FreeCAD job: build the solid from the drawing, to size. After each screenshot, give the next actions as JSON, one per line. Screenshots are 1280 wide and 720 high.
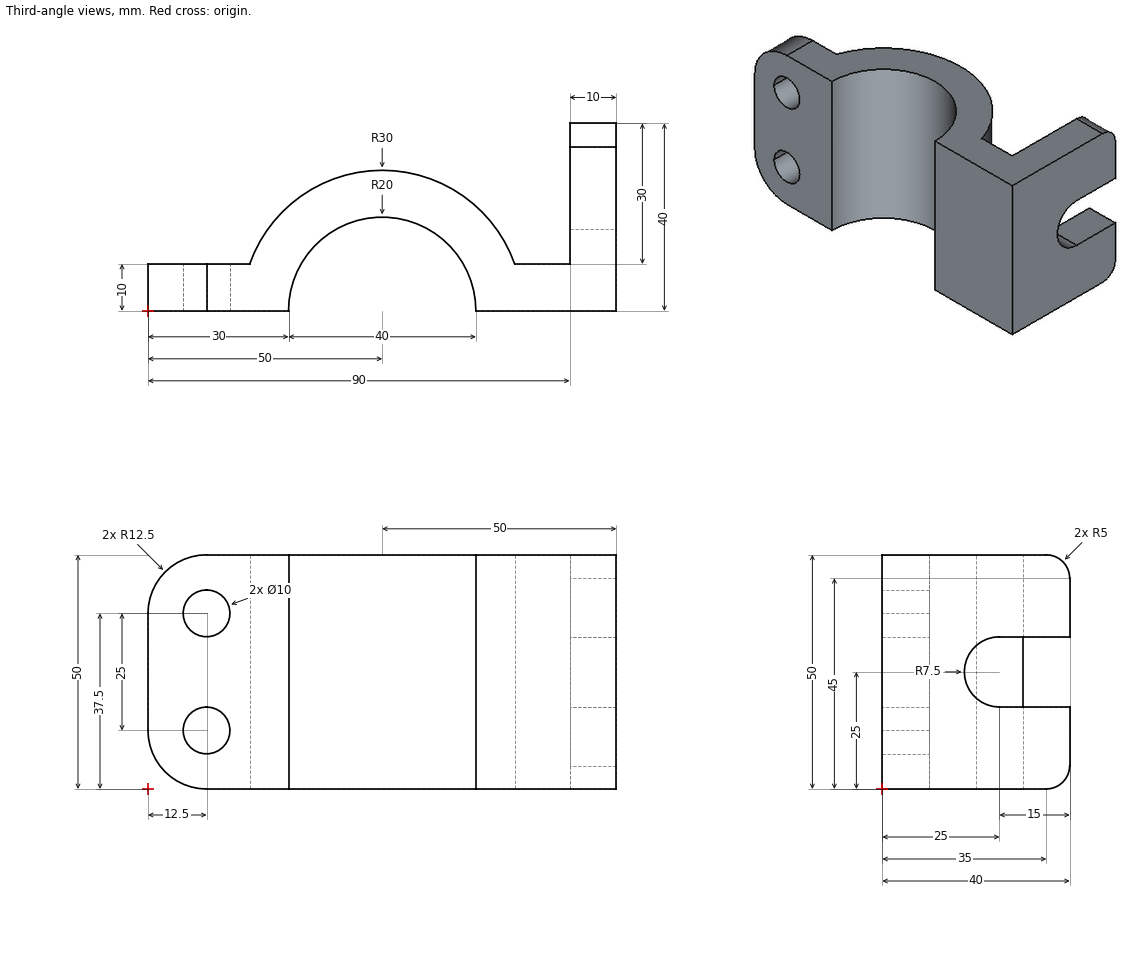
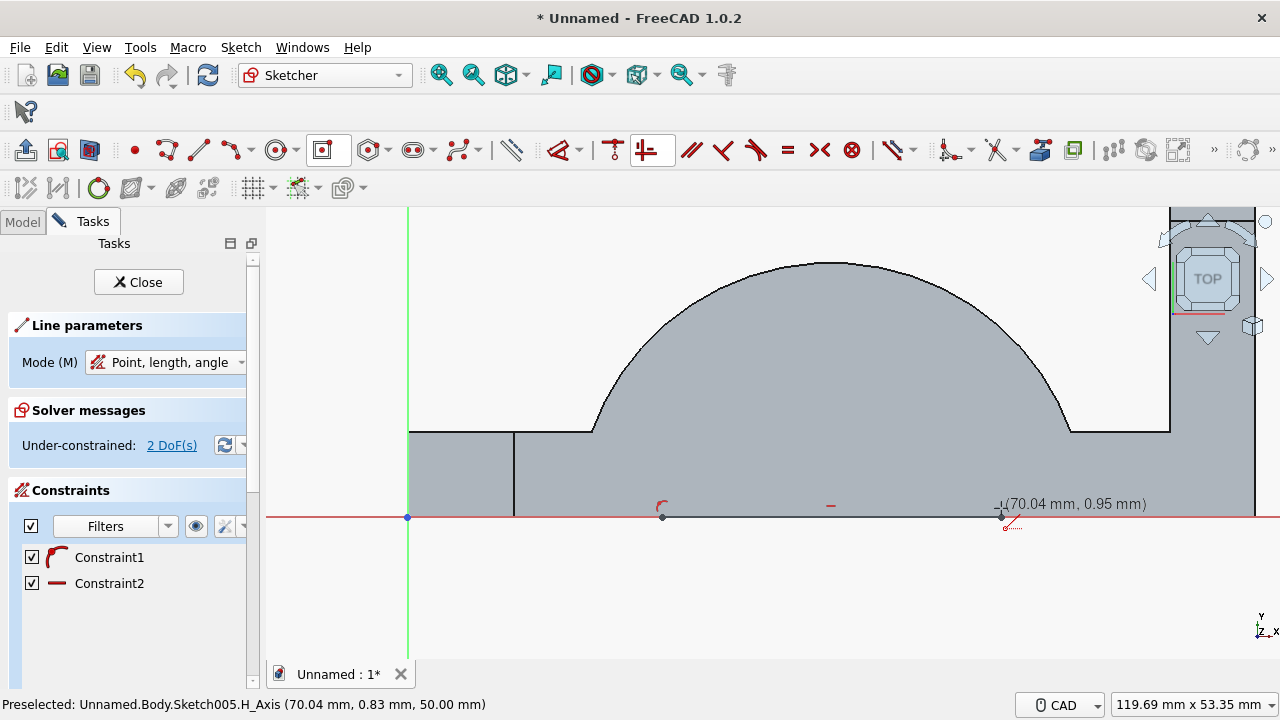
{"action": "left_click", "coordinate": [232, 150]}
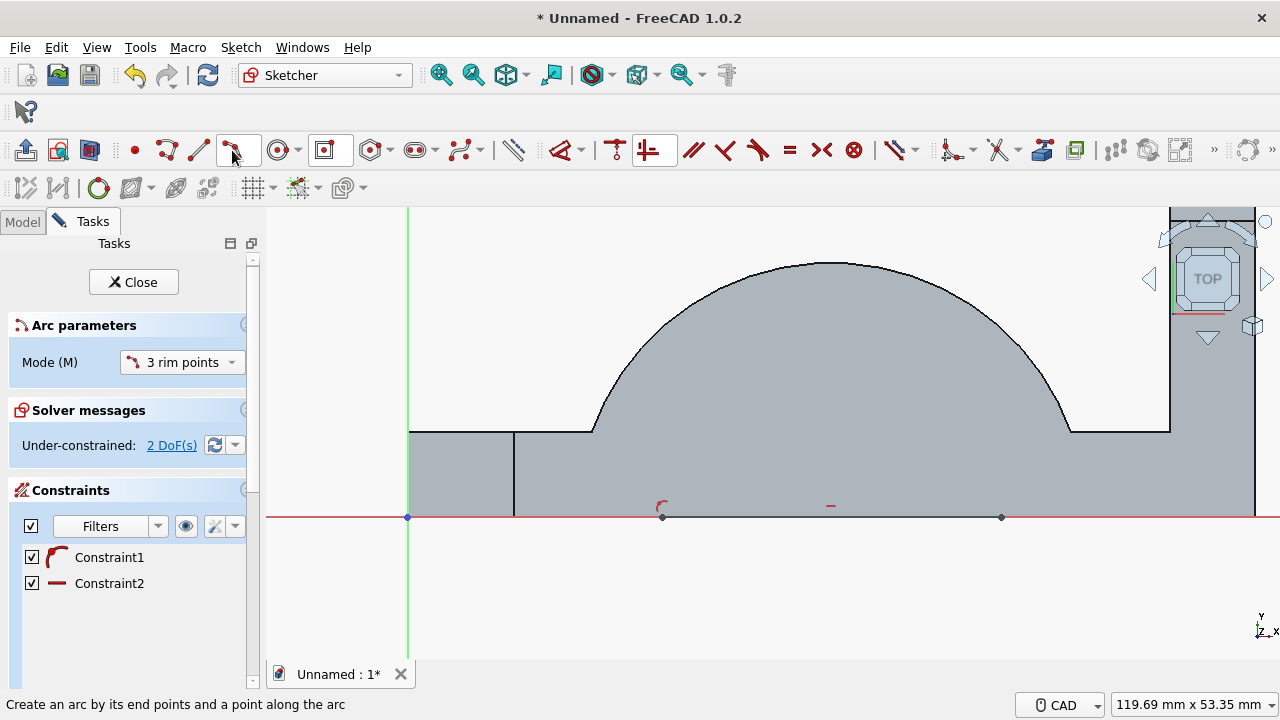
{"action": "left_click", "coordinate": [1001, 508]}
{"action": "left_click", "coordinate": [662, 517]}
{"action": "left_click", "coordinate": [831, 348]}
{"action": "key", "text": "Escape"}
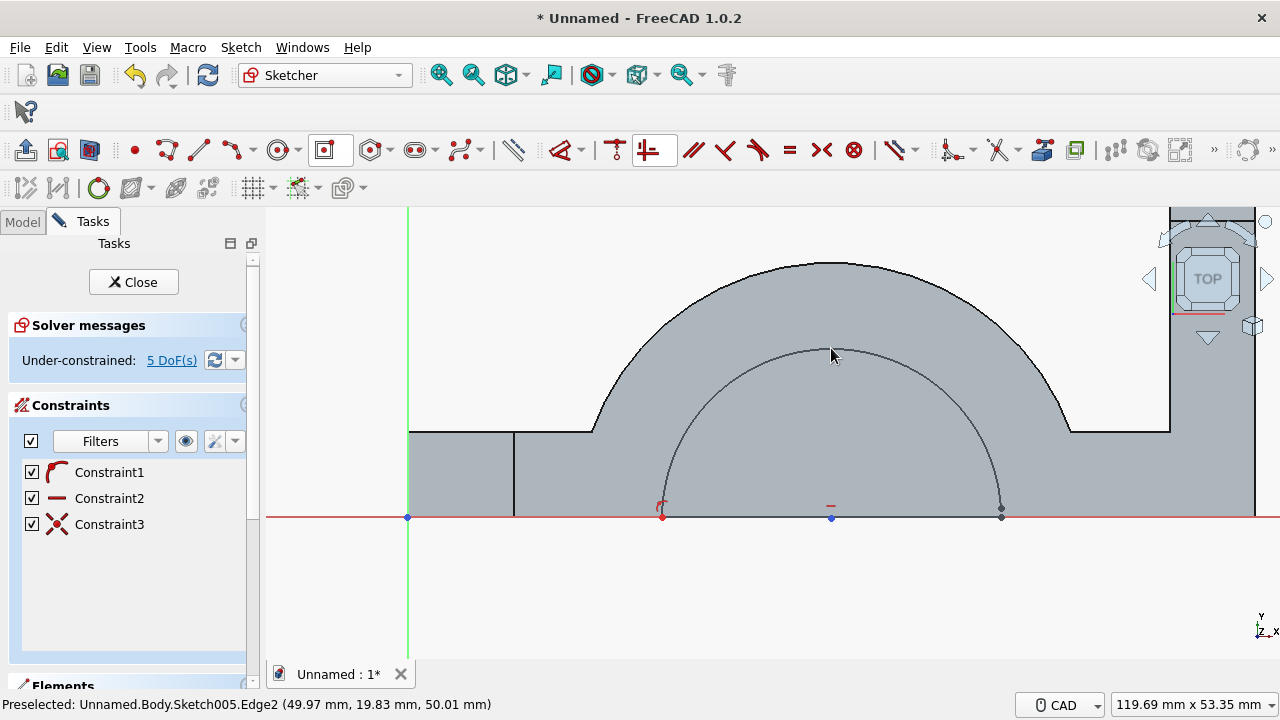
{"action": "left_click", "coordinate": [832, 519]}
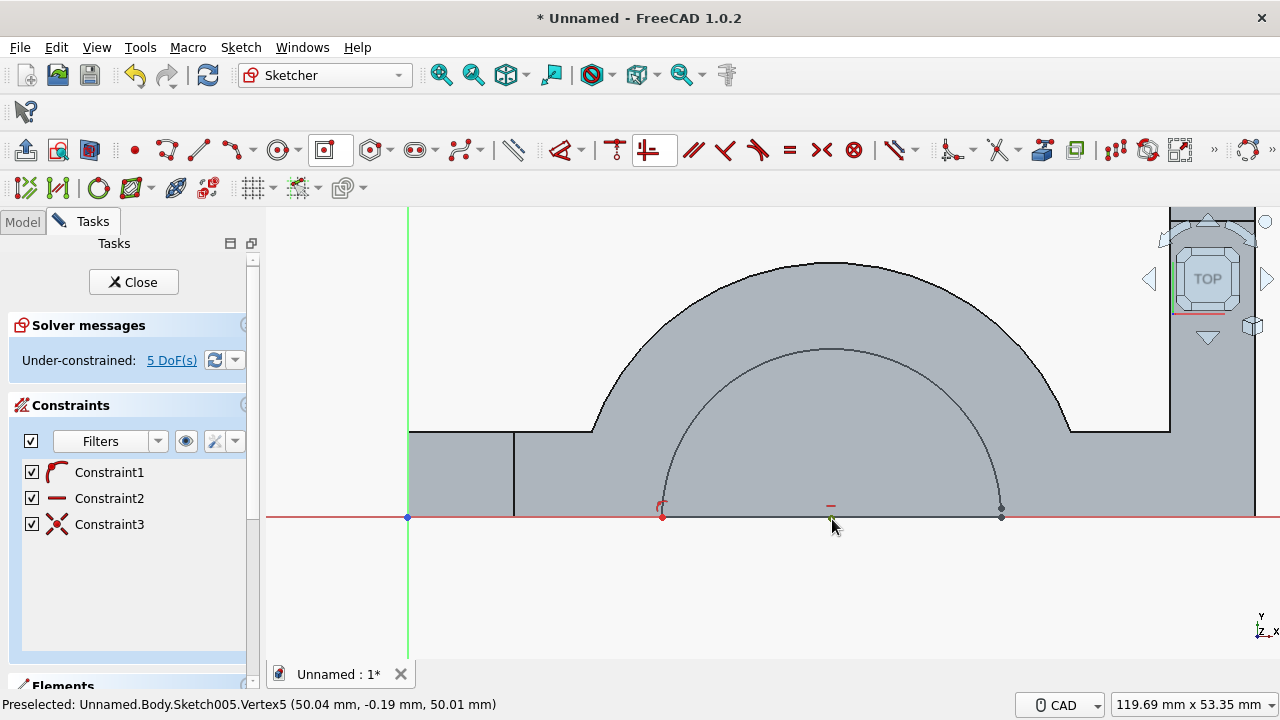
{"action": "left_click", "coordinate": [353, 517]}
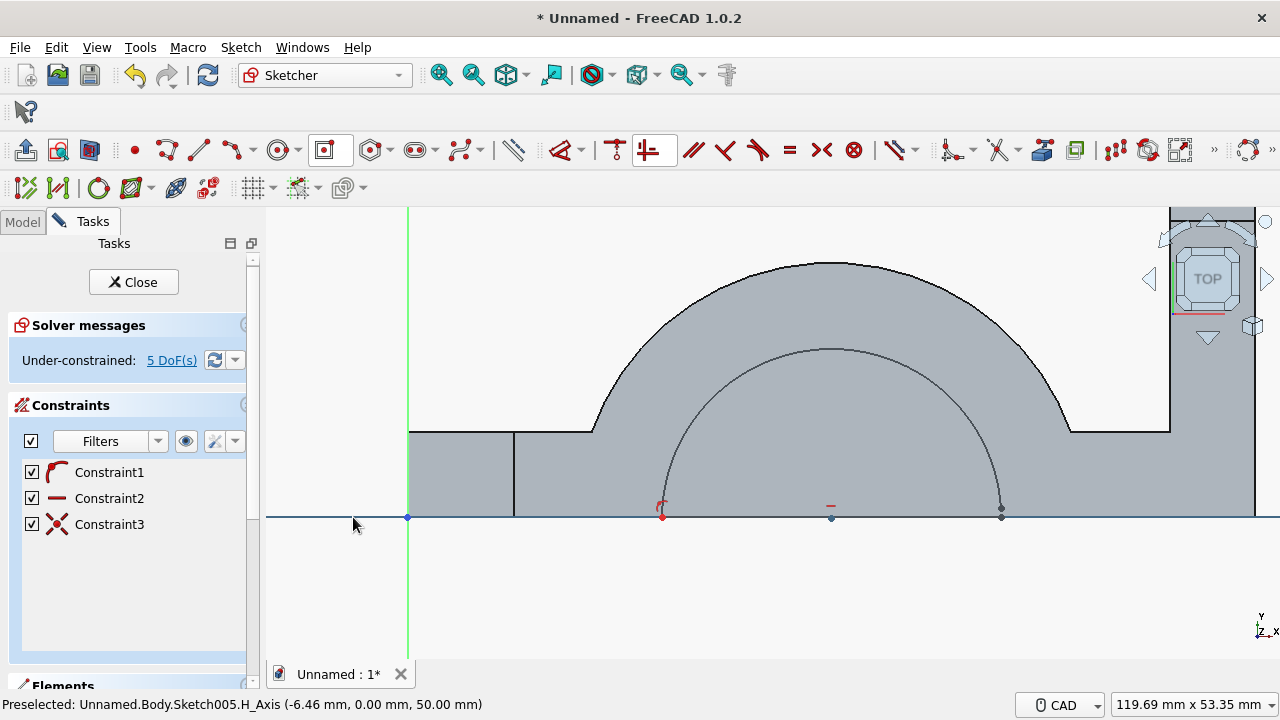
{"action": "left_click", "coordinate": [616, 150]}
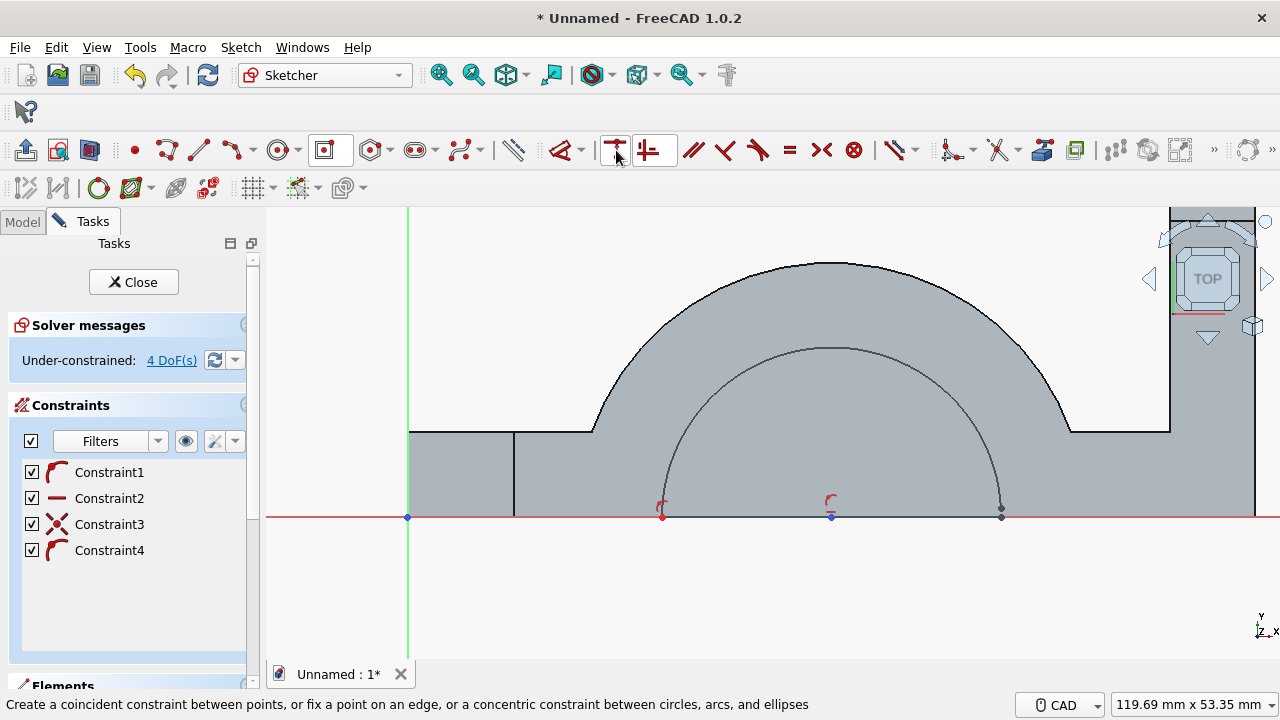
{"action": "left_click", "coordinate": [560, 150]}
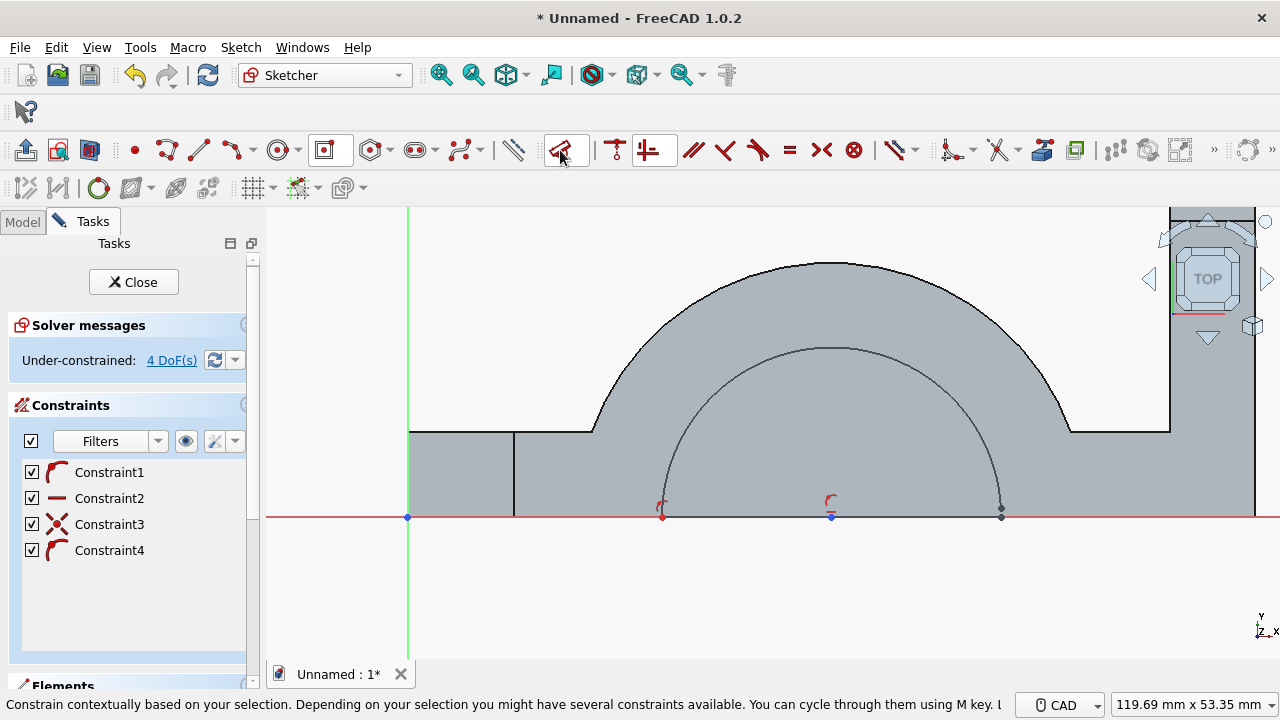
{"action": "left_click", "coordinate": [927, 377]}
{"action": "left_click", "coordinate": [945, 351]}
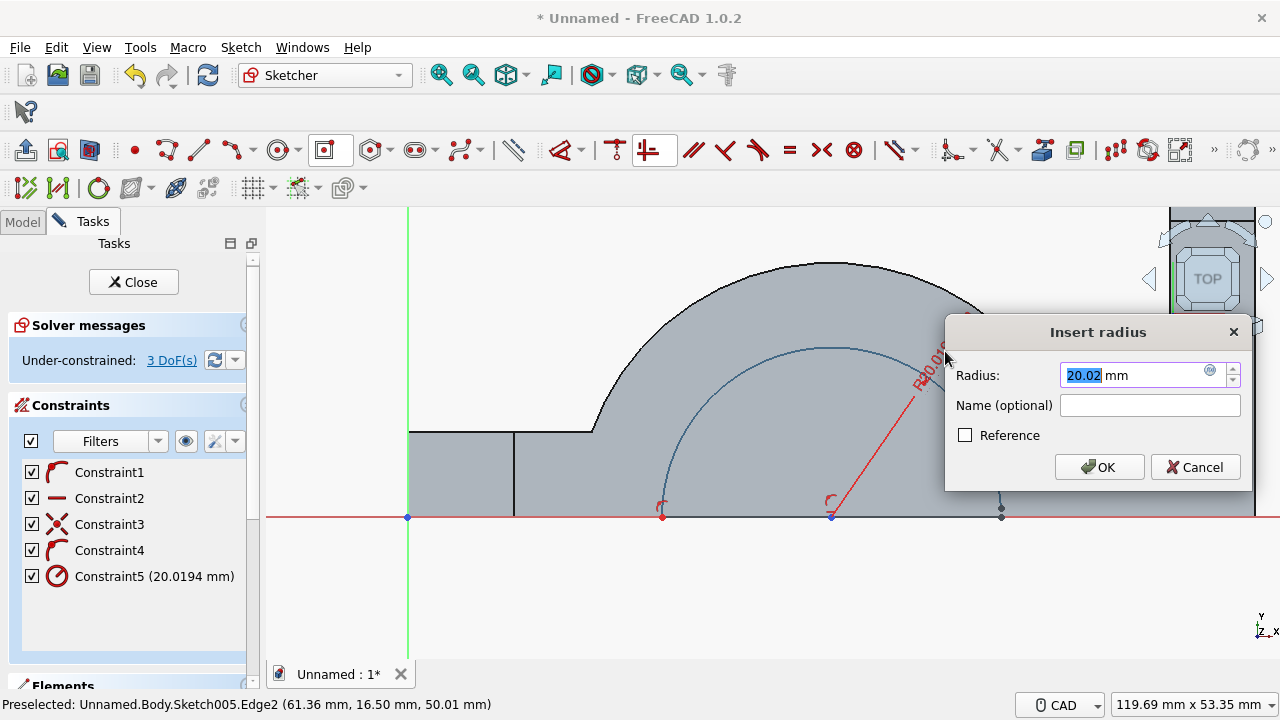
{"action": "type", "text": "20"}
{"action": "key", "text": "Return"}
{"action": "key", "text": "Escape"}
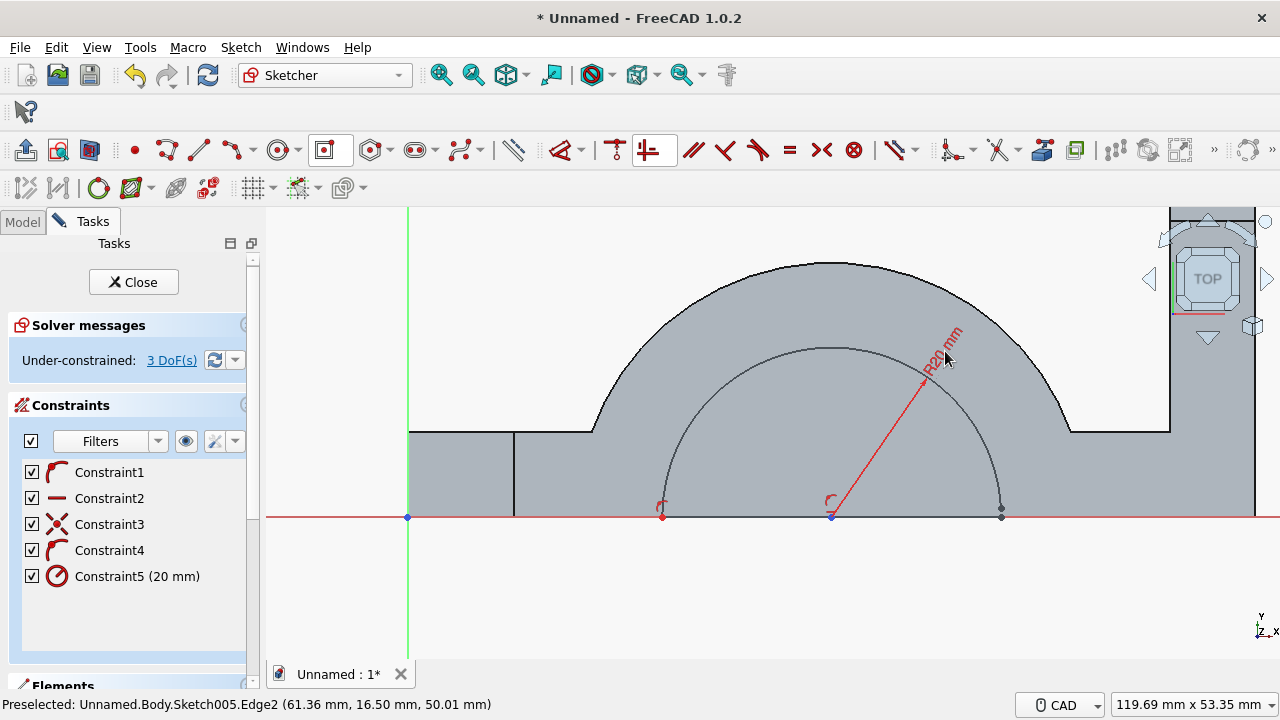
{"action": "left_click", "coordinate": [1001, 509]}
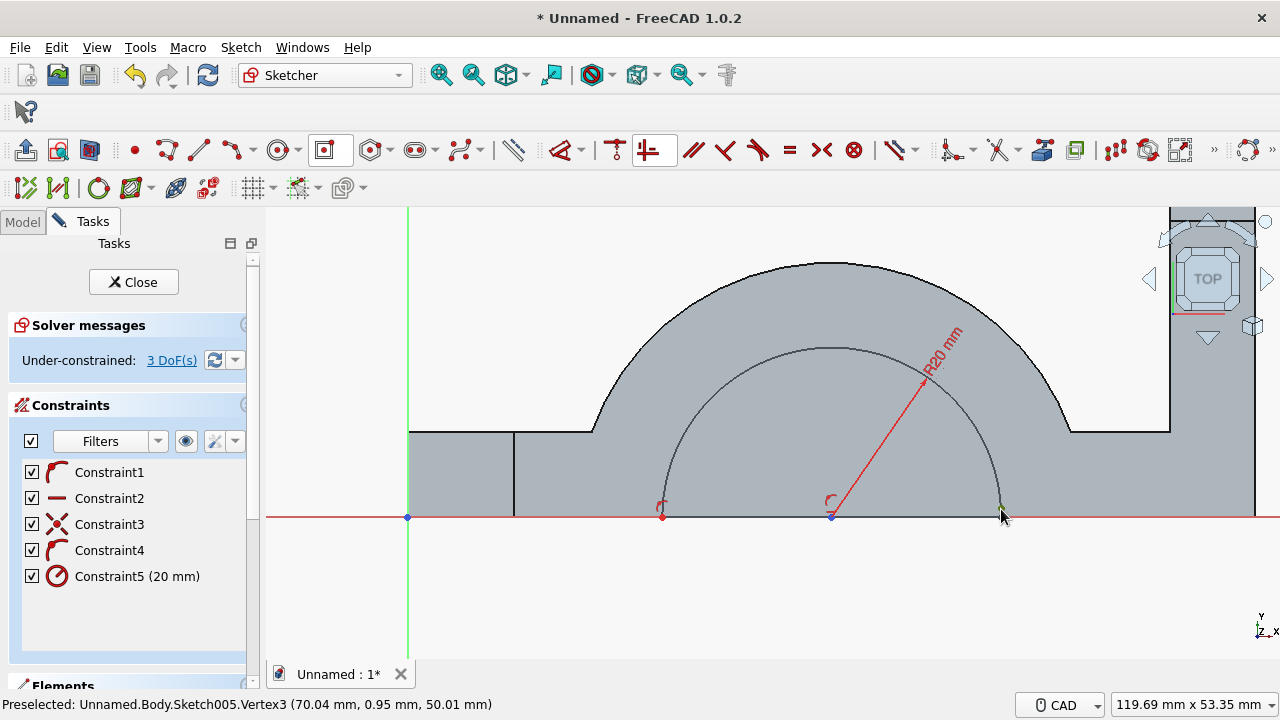
{"action": "left_click", "coordinate": [353, 517]}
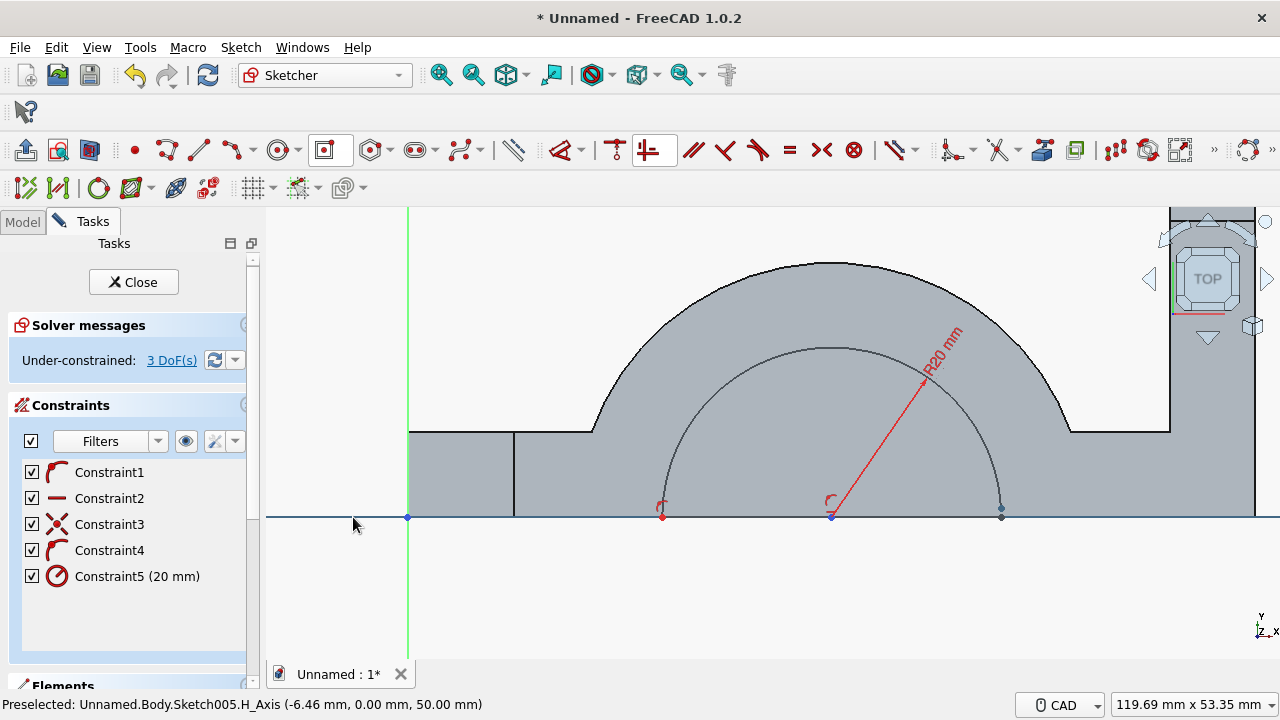
{"action": "left_click", "coordinate": [616, 150]}